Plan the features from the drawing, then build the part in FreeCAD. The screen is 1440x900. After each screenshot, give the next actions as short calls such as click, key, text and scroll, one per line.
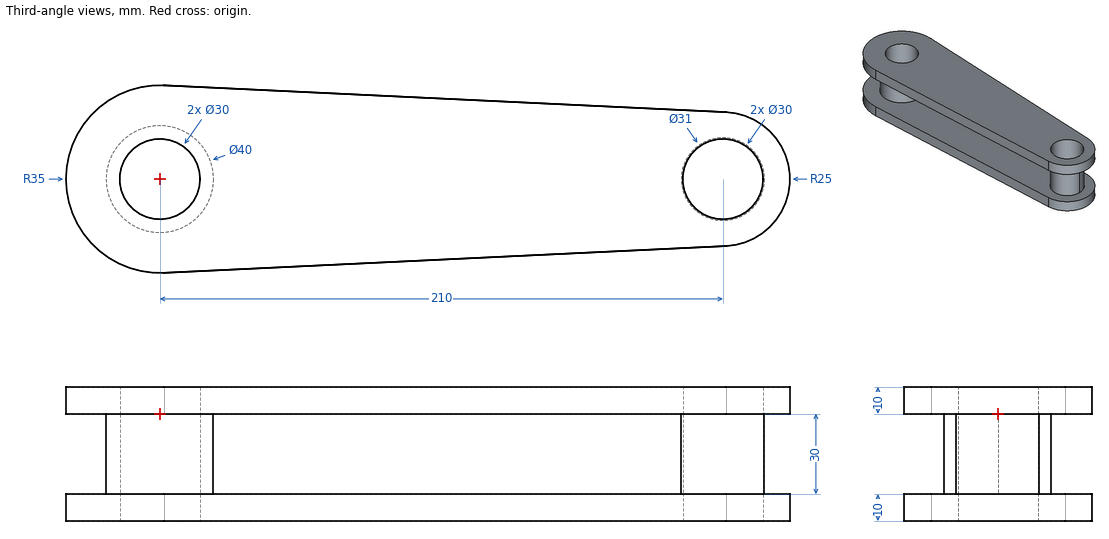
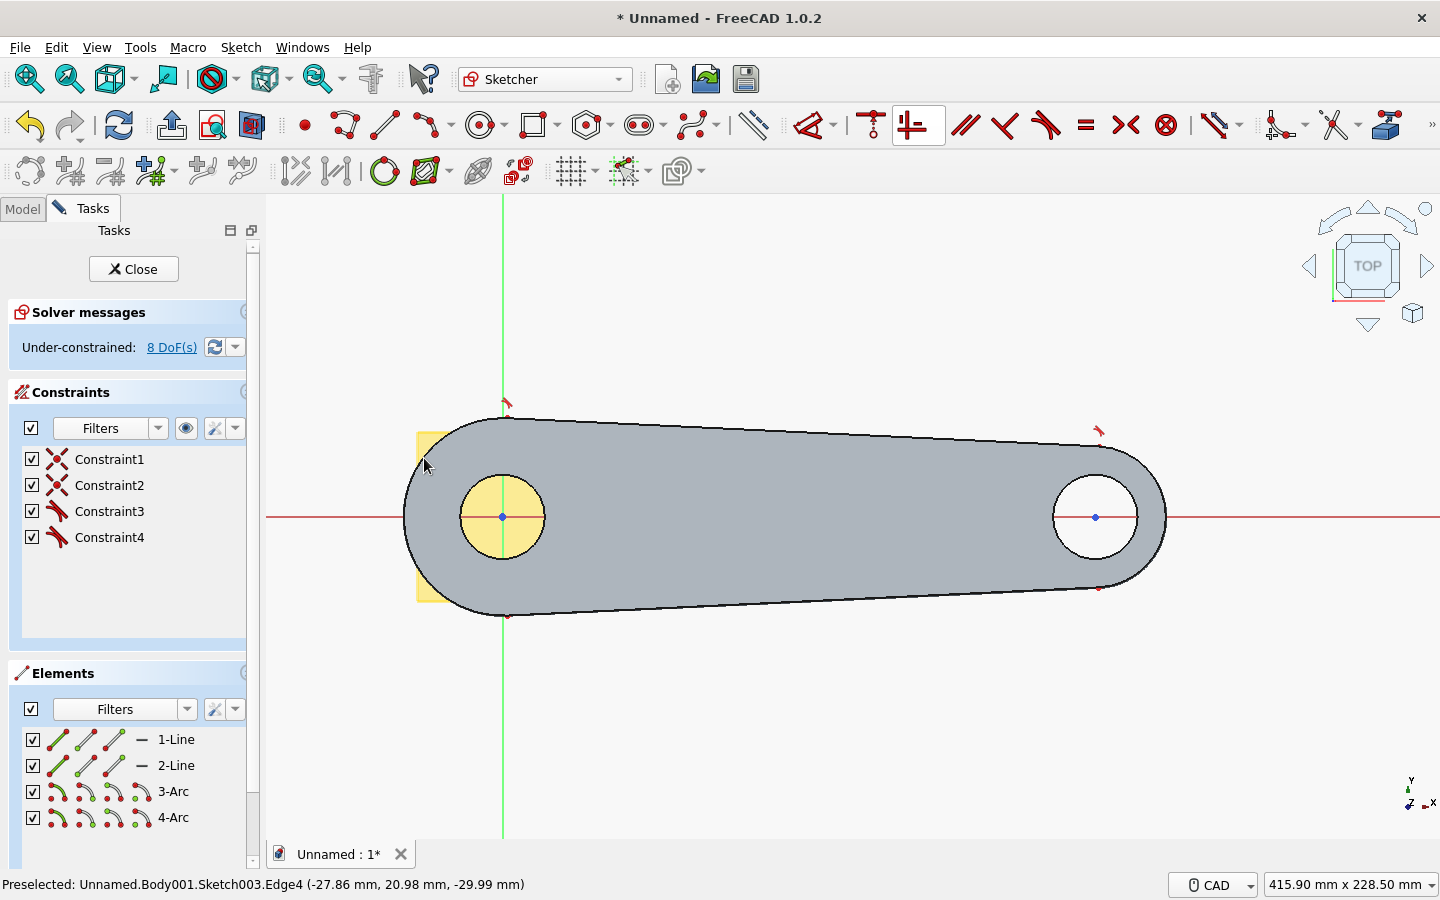
click(921, 596)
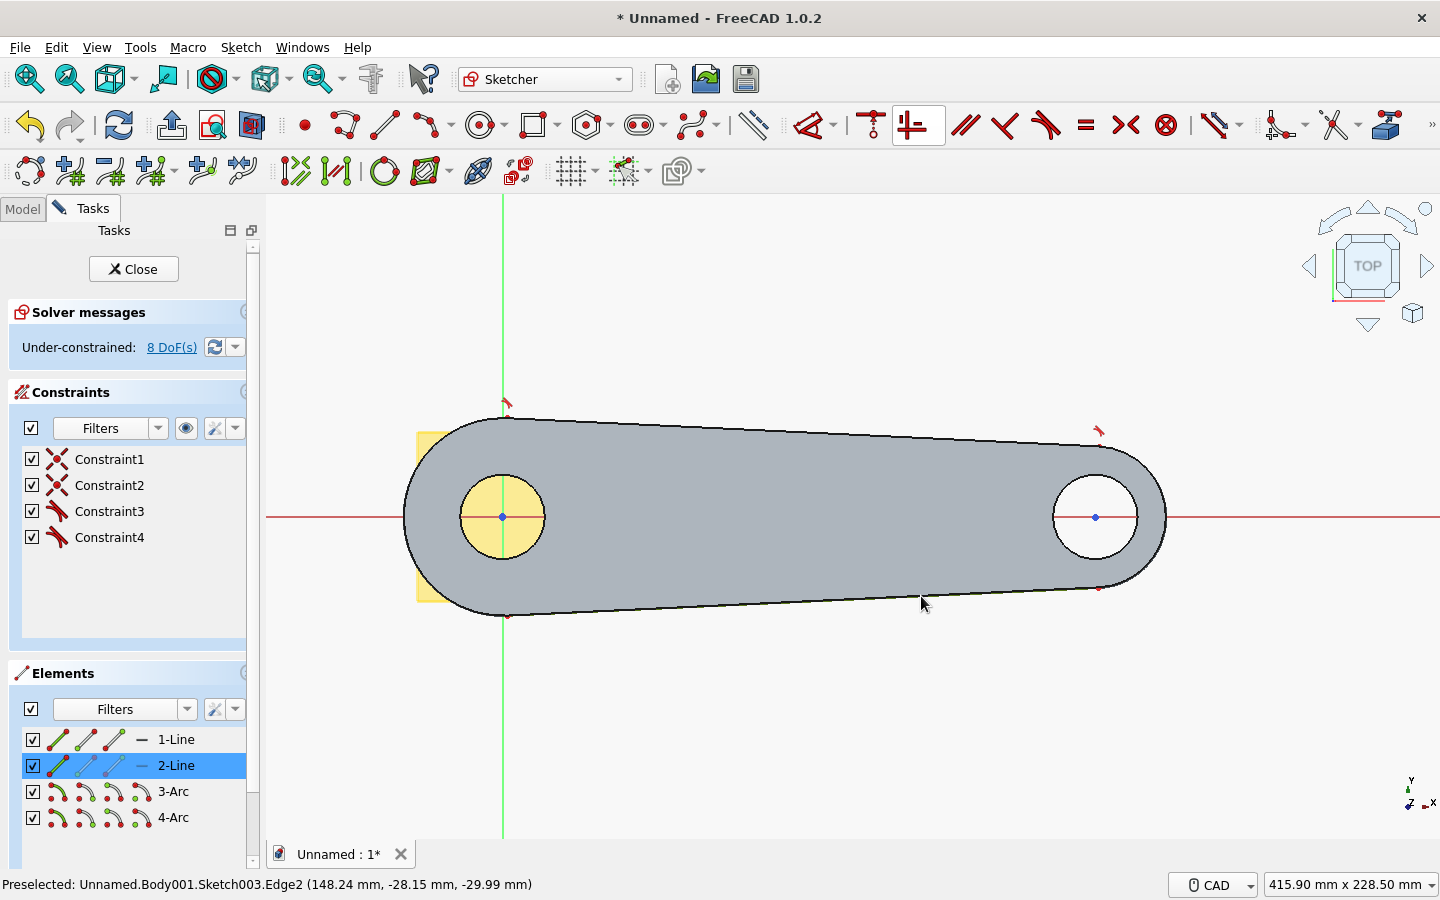
click(1154, 558)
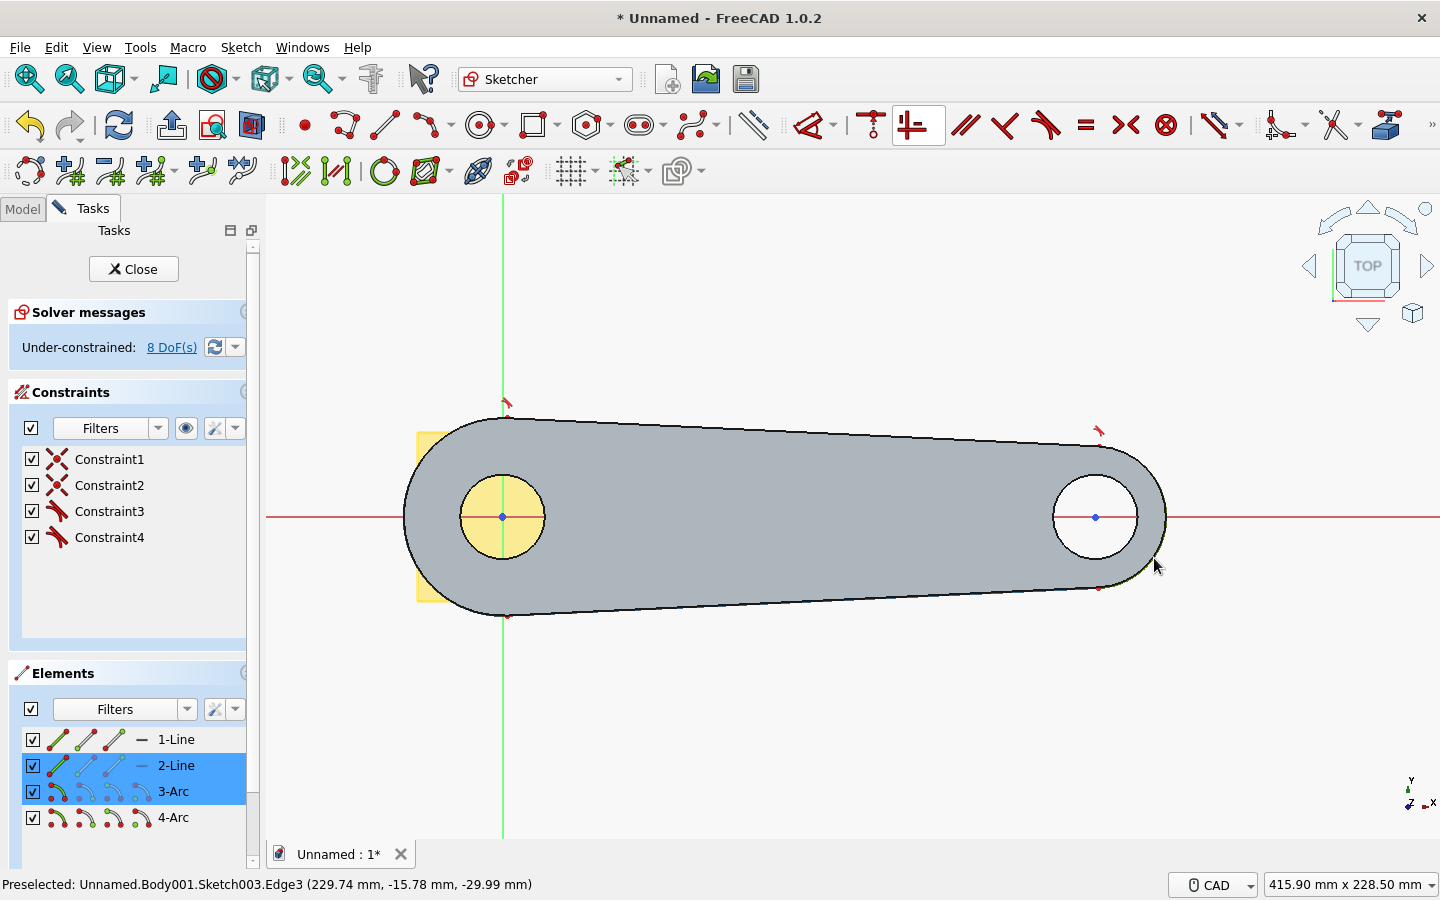
click(1046, 126)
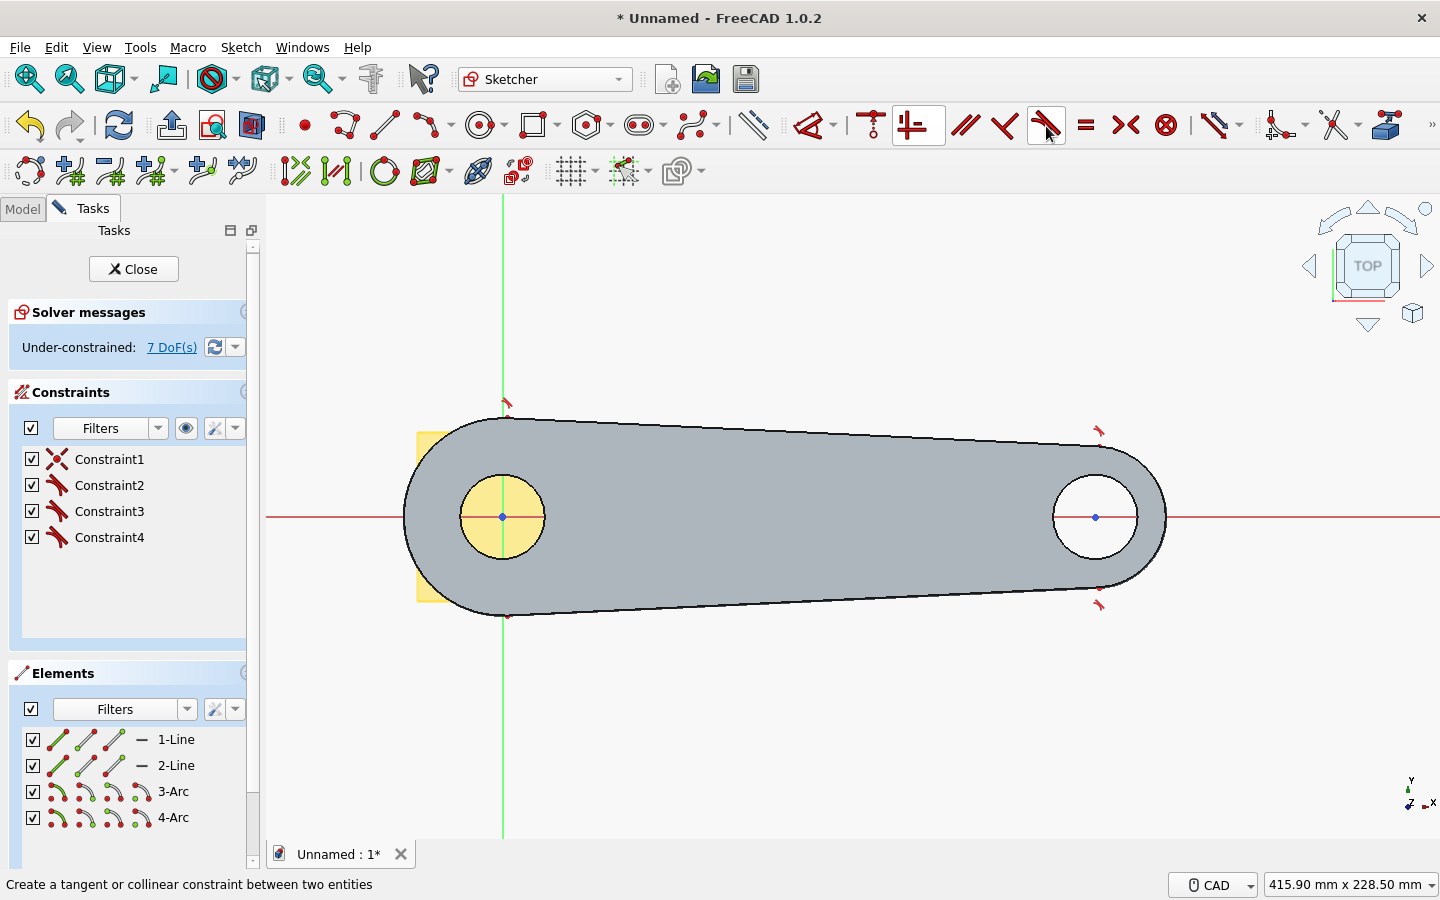
click(922, 596)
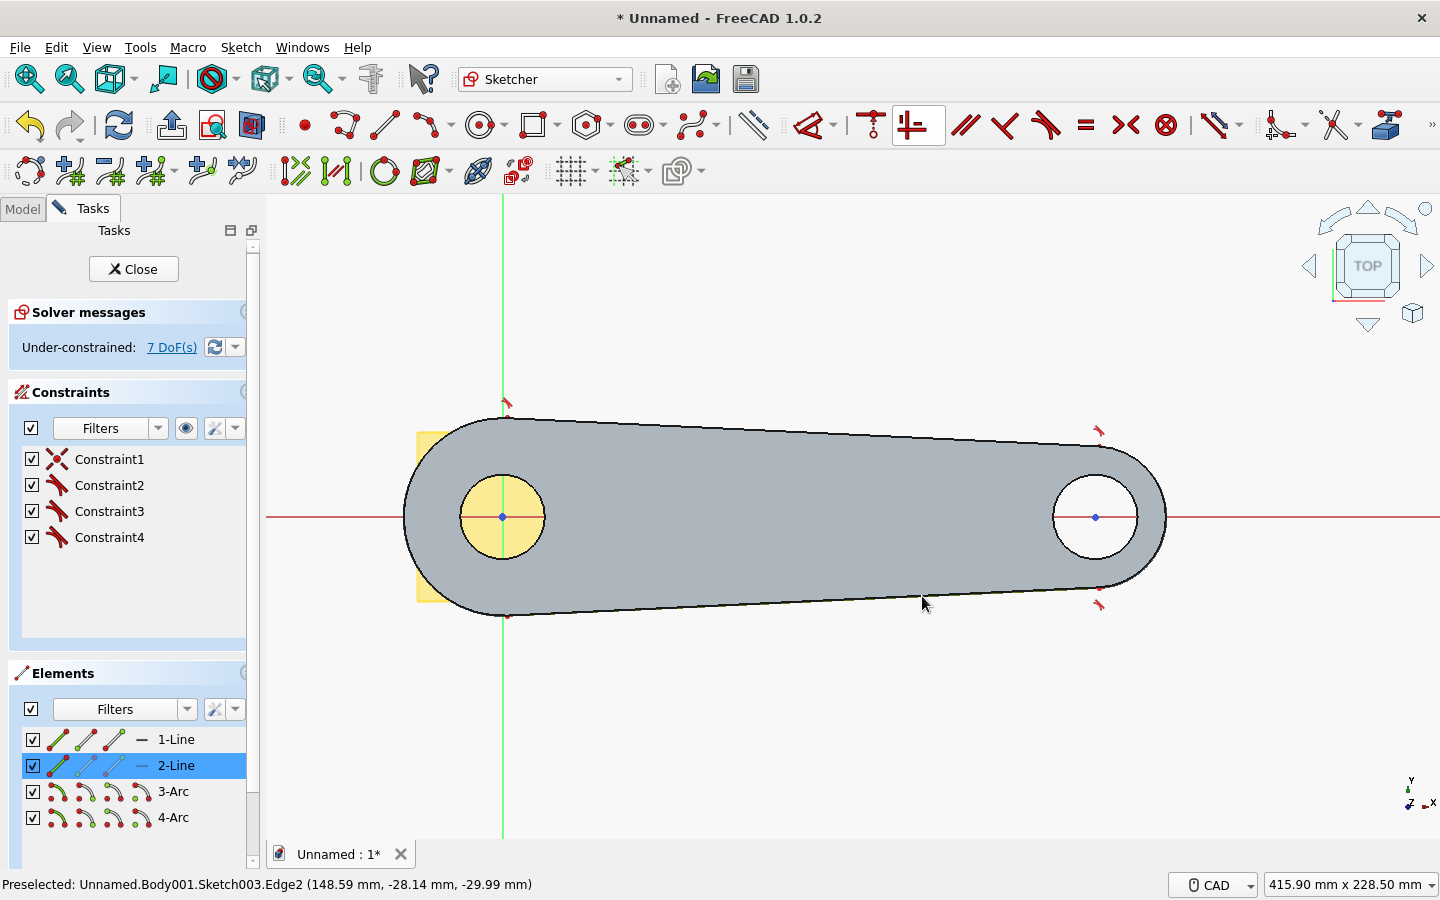
click(424, 458)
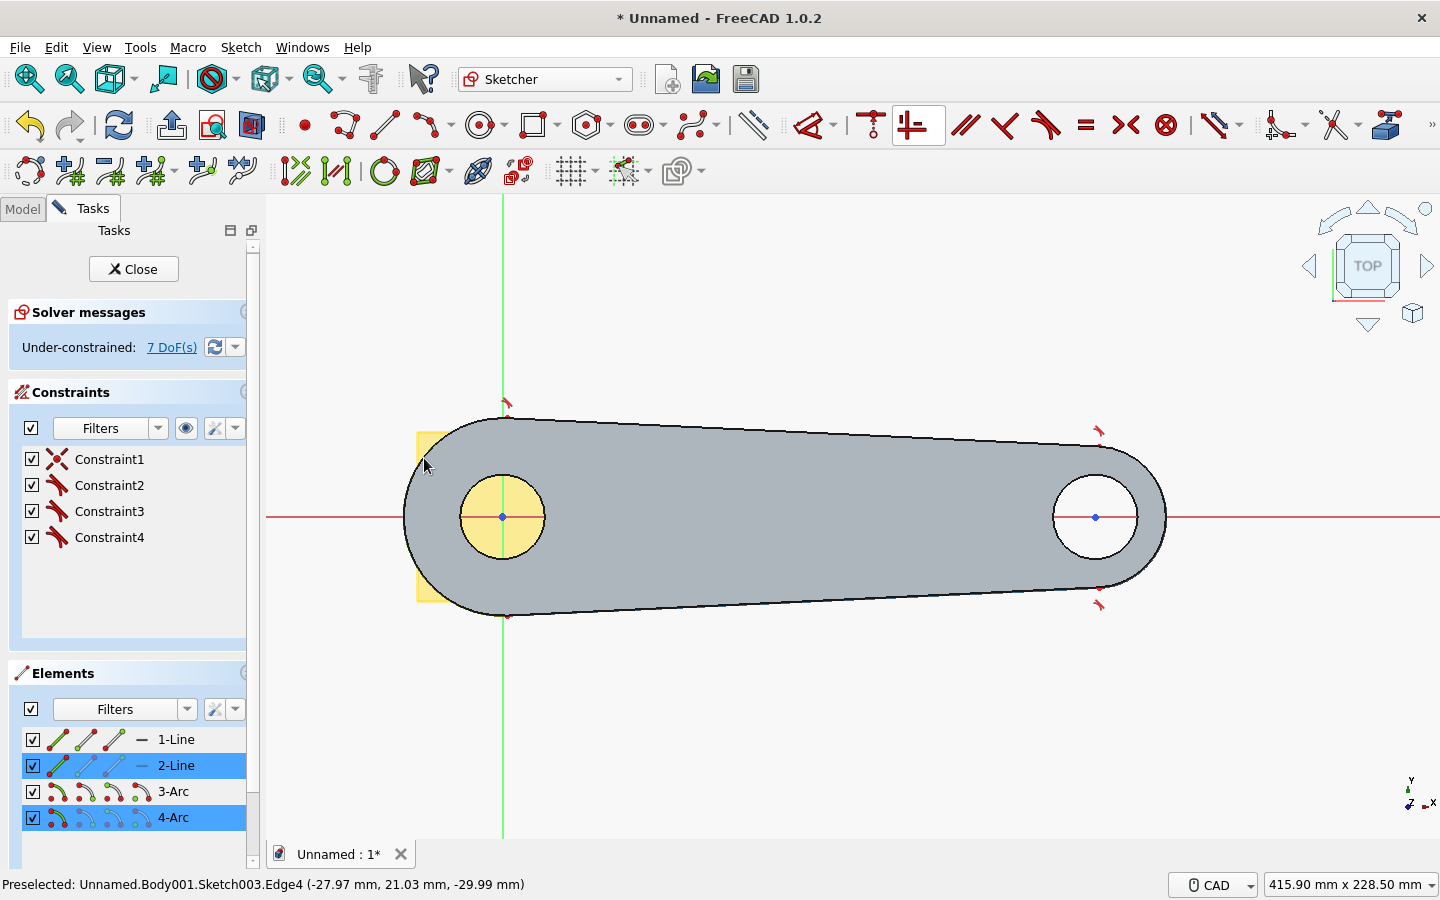
key(t)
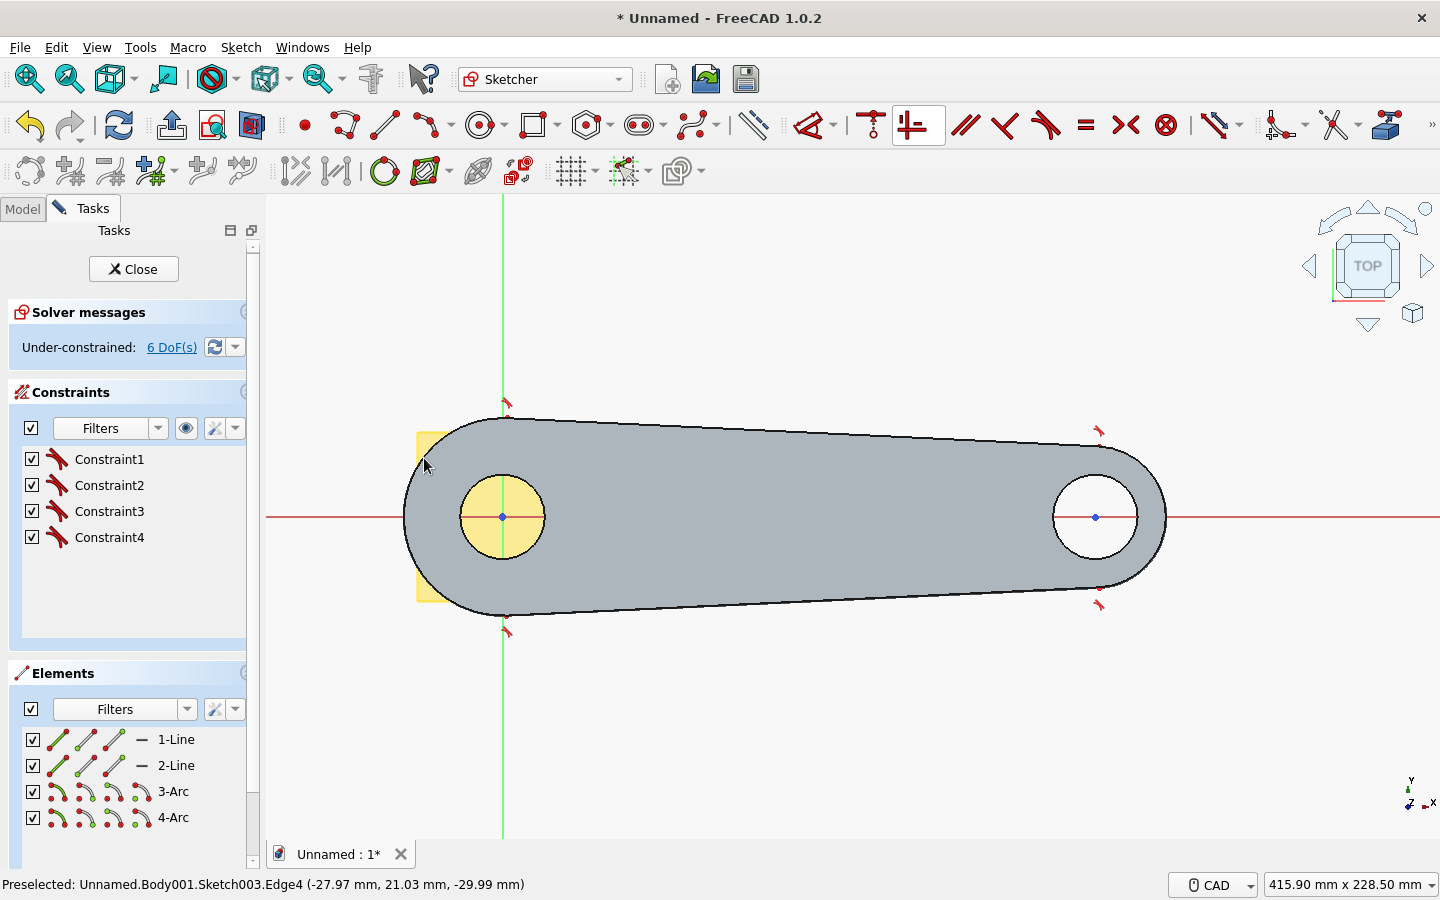
drag(492, 507, 513, 527)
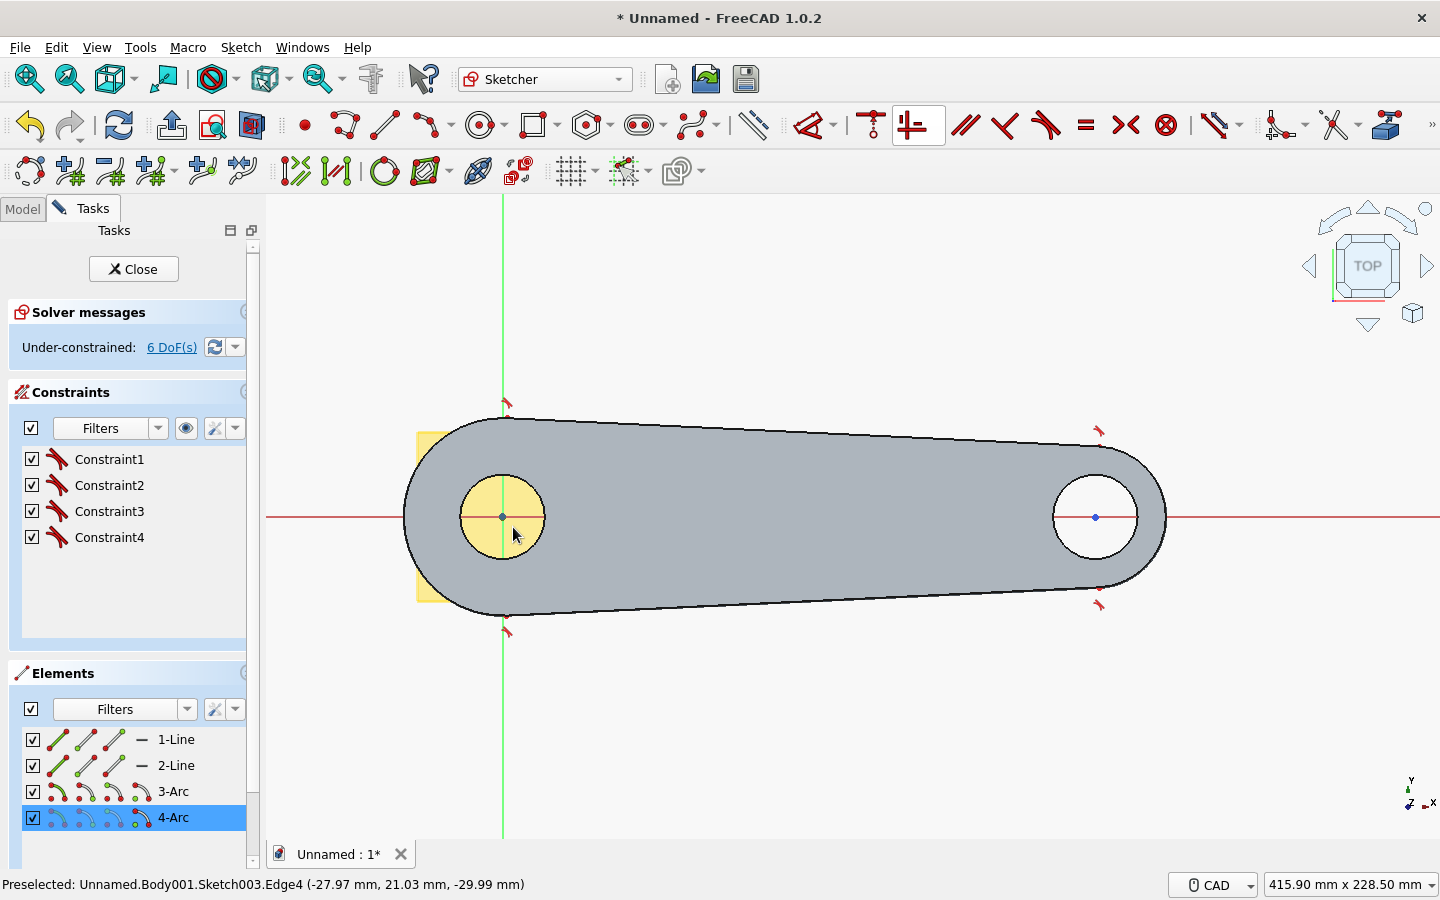
key(c)